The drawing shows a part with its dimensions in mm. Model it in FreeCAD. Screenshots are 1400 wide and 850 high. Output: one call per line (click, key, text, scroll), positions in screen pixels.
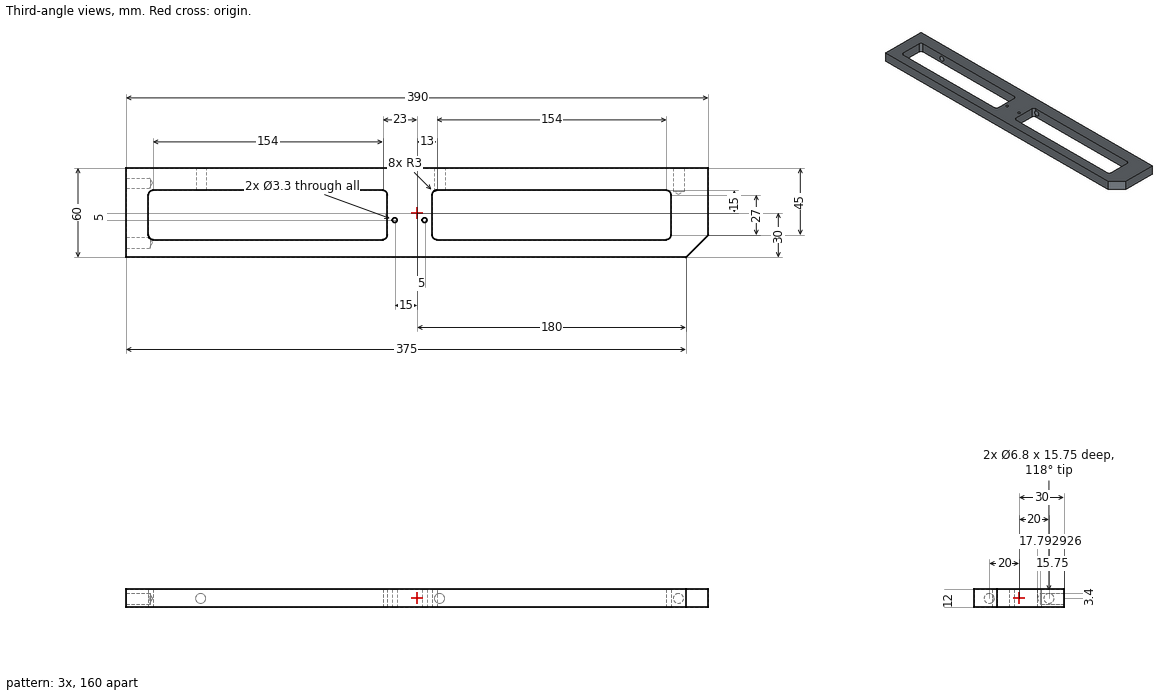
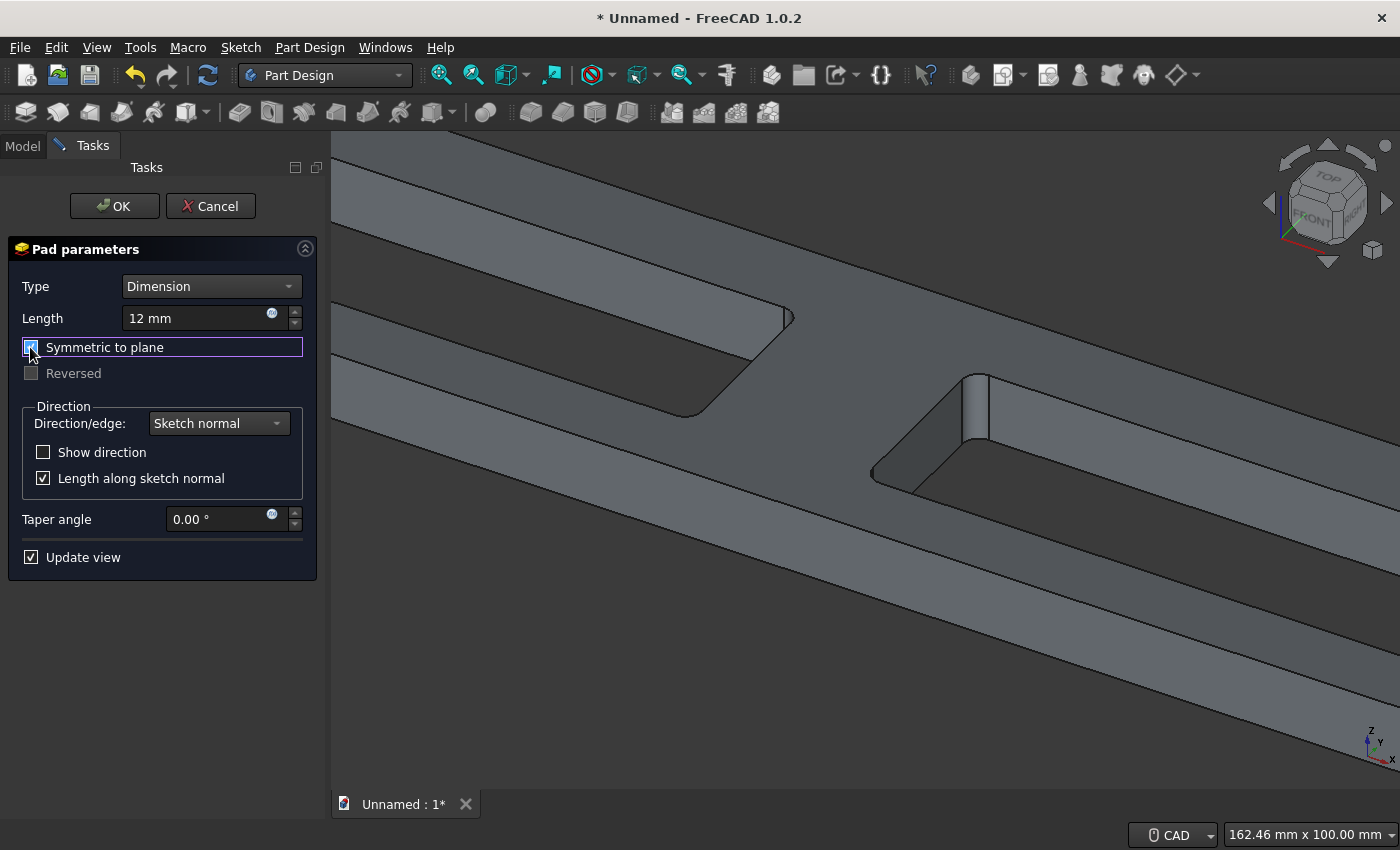
click(115, 206)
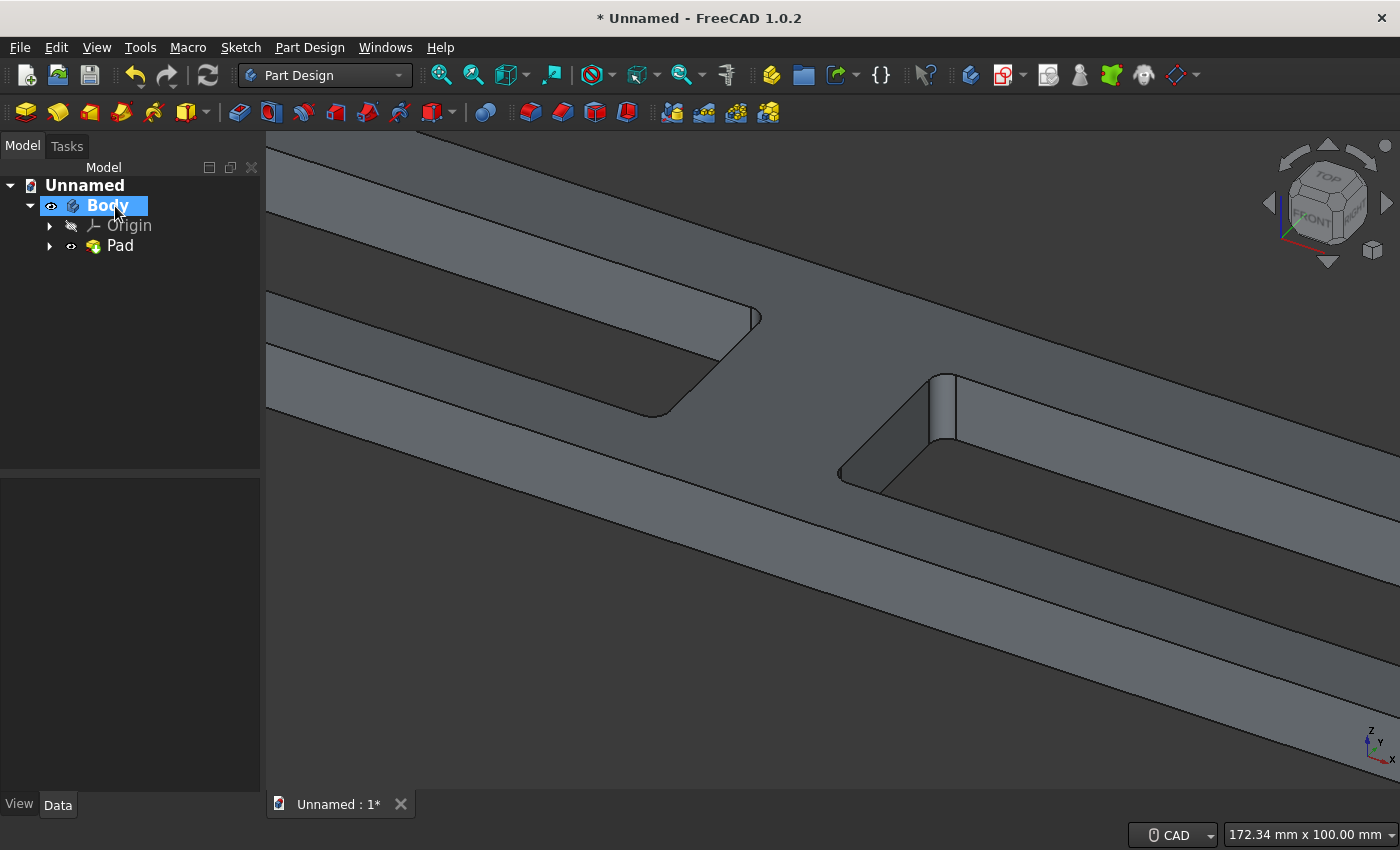
key(v)
key(f)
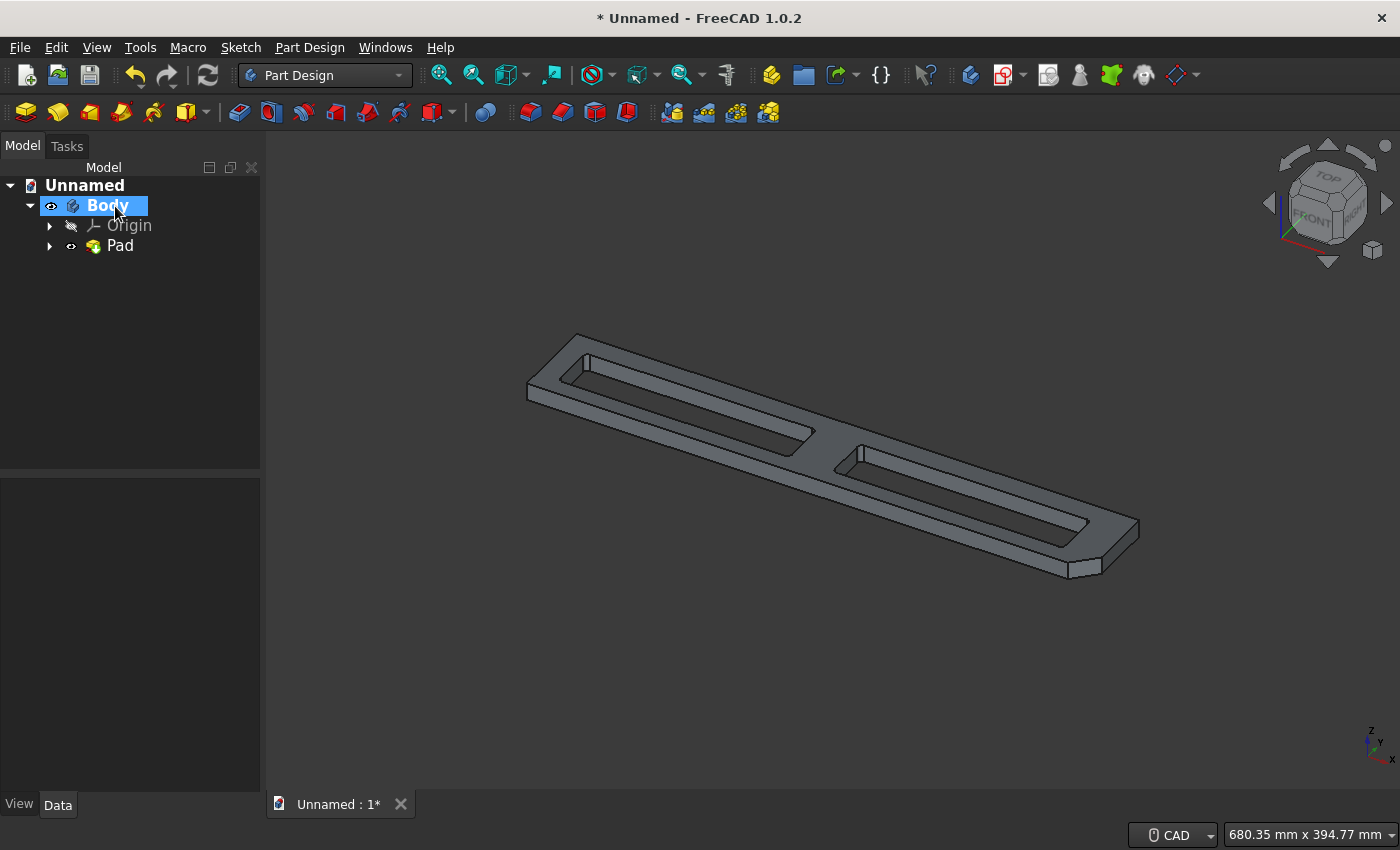
key(6)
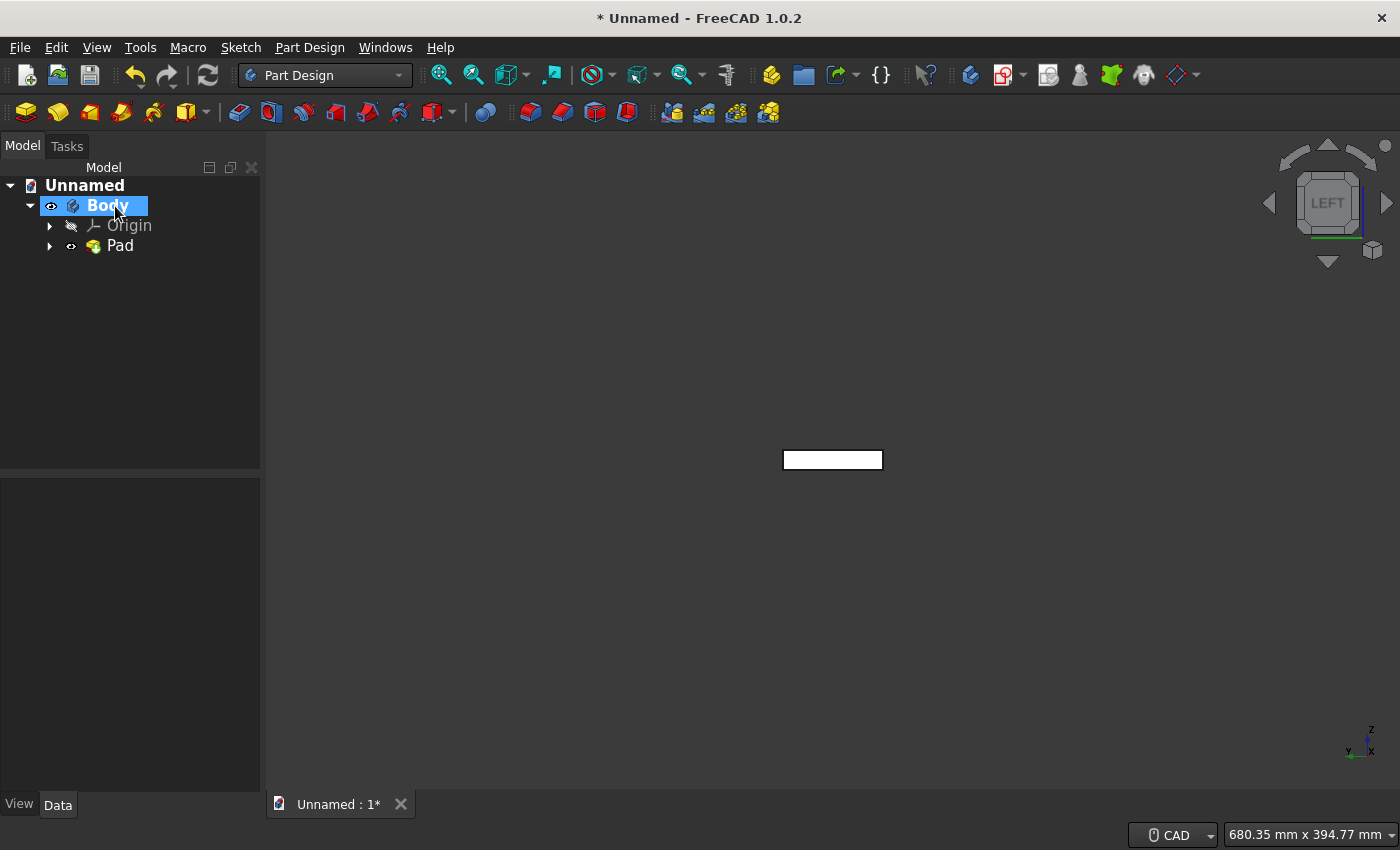
key(v)
key(f)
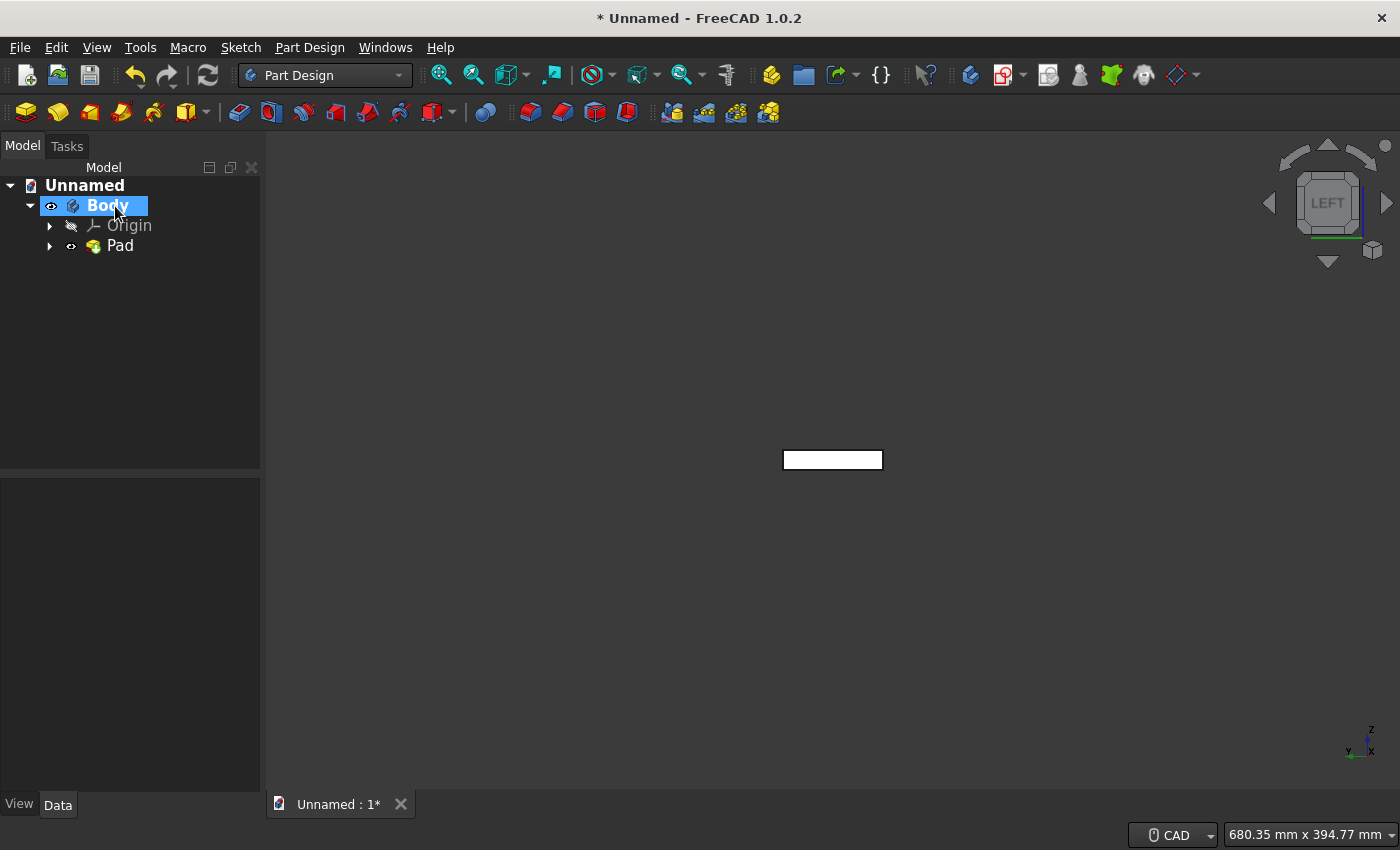
click(804, 459)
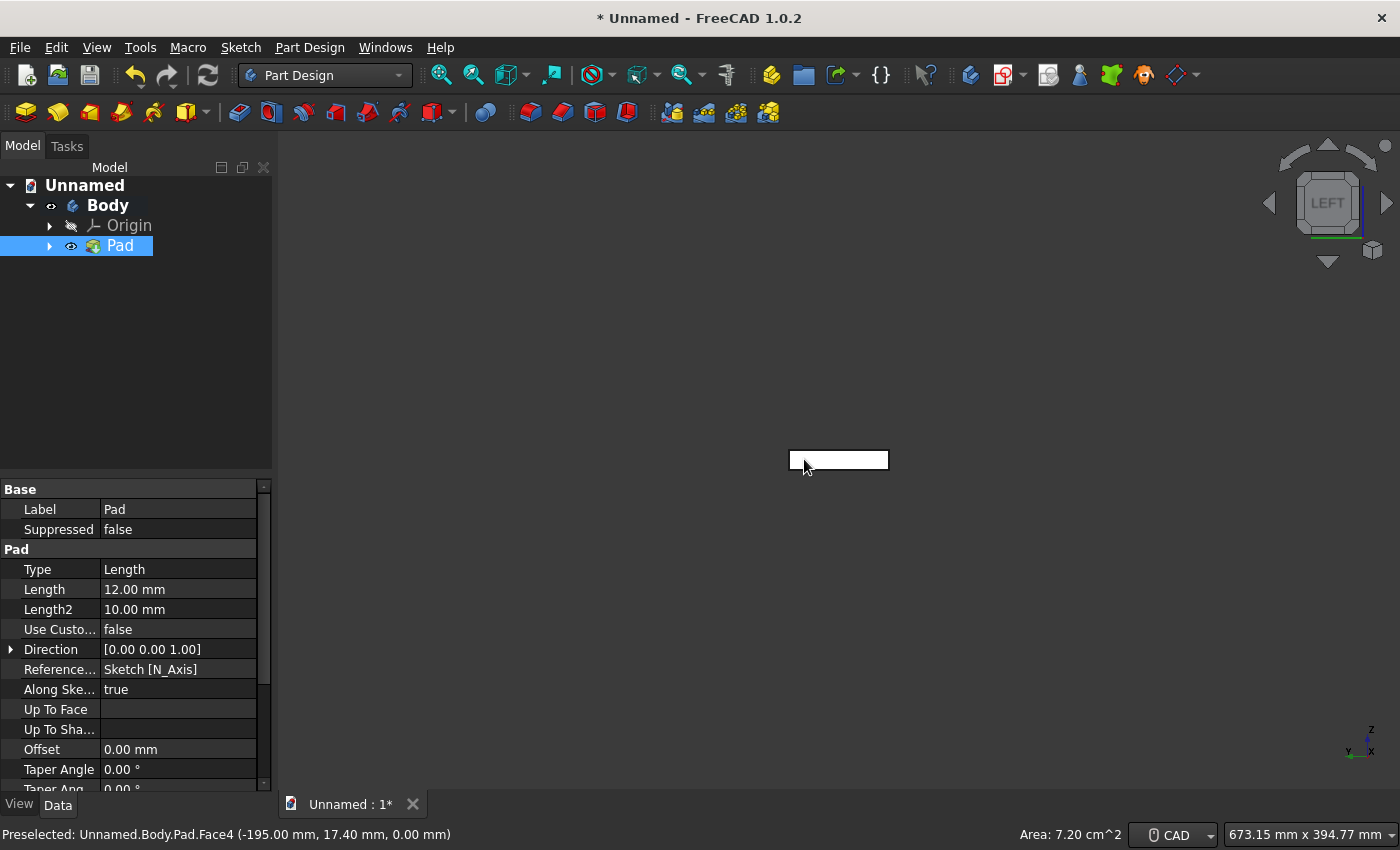
click(1004, 76)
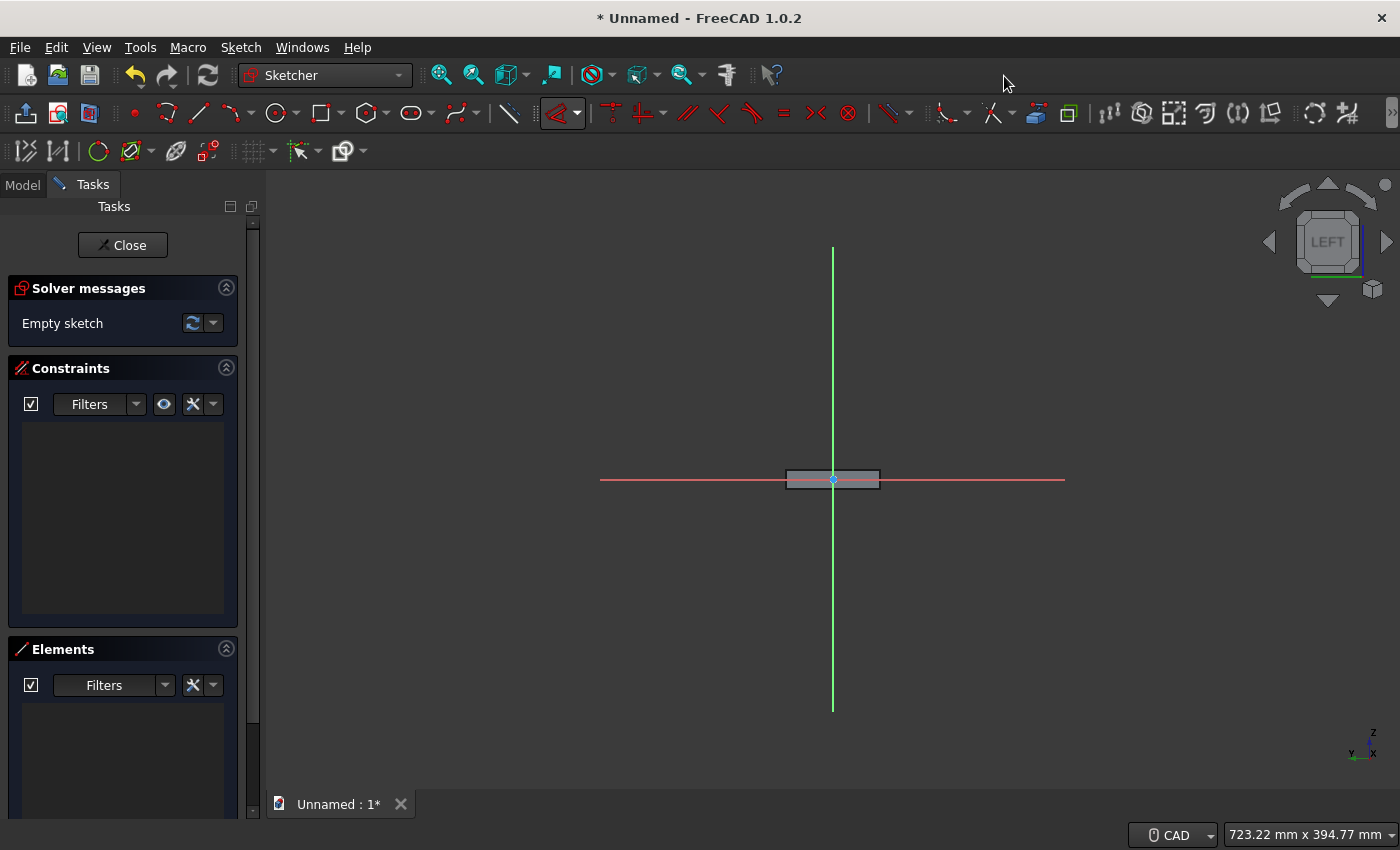
scroll(842, 479, up, 11)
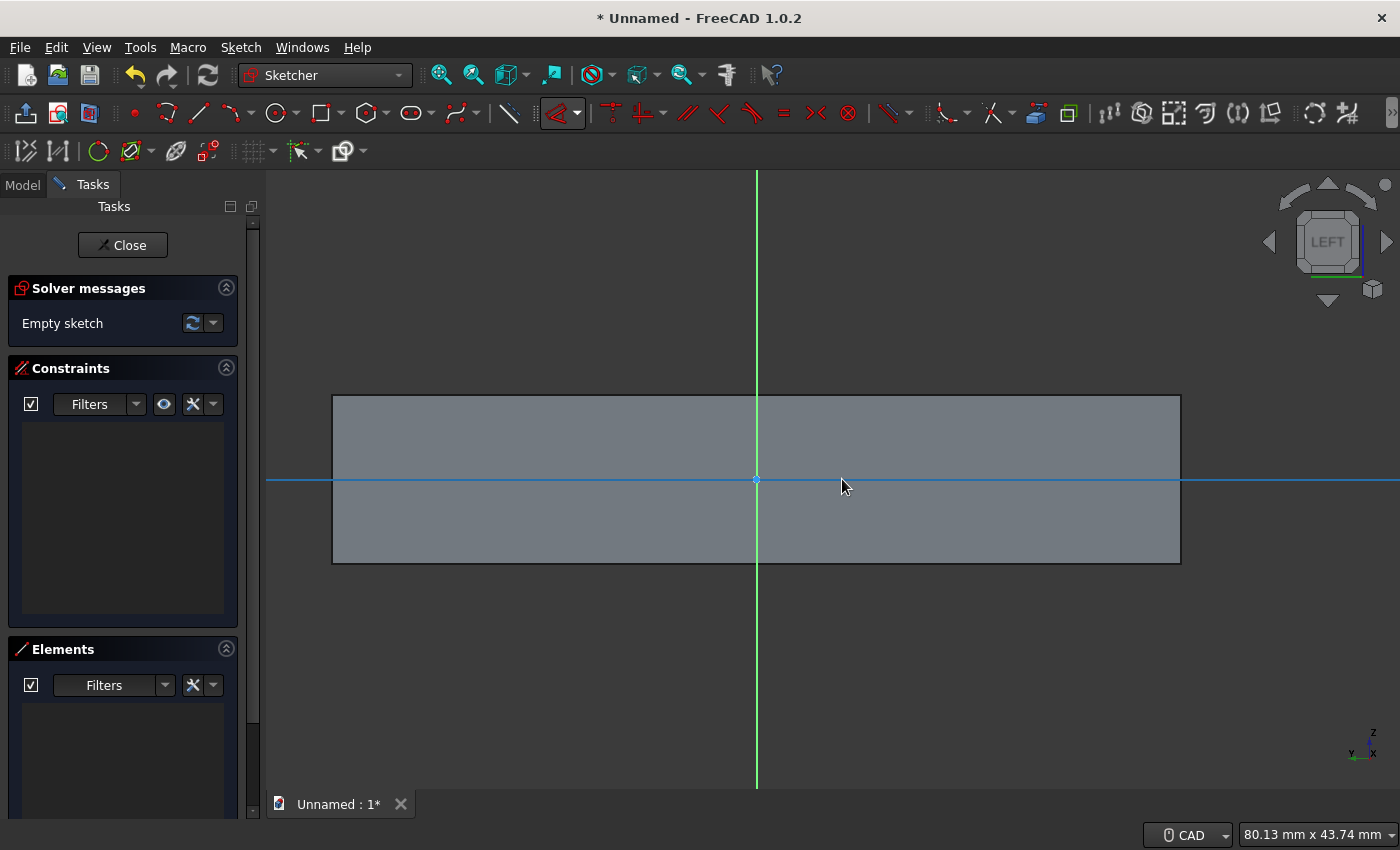
click(276, 114)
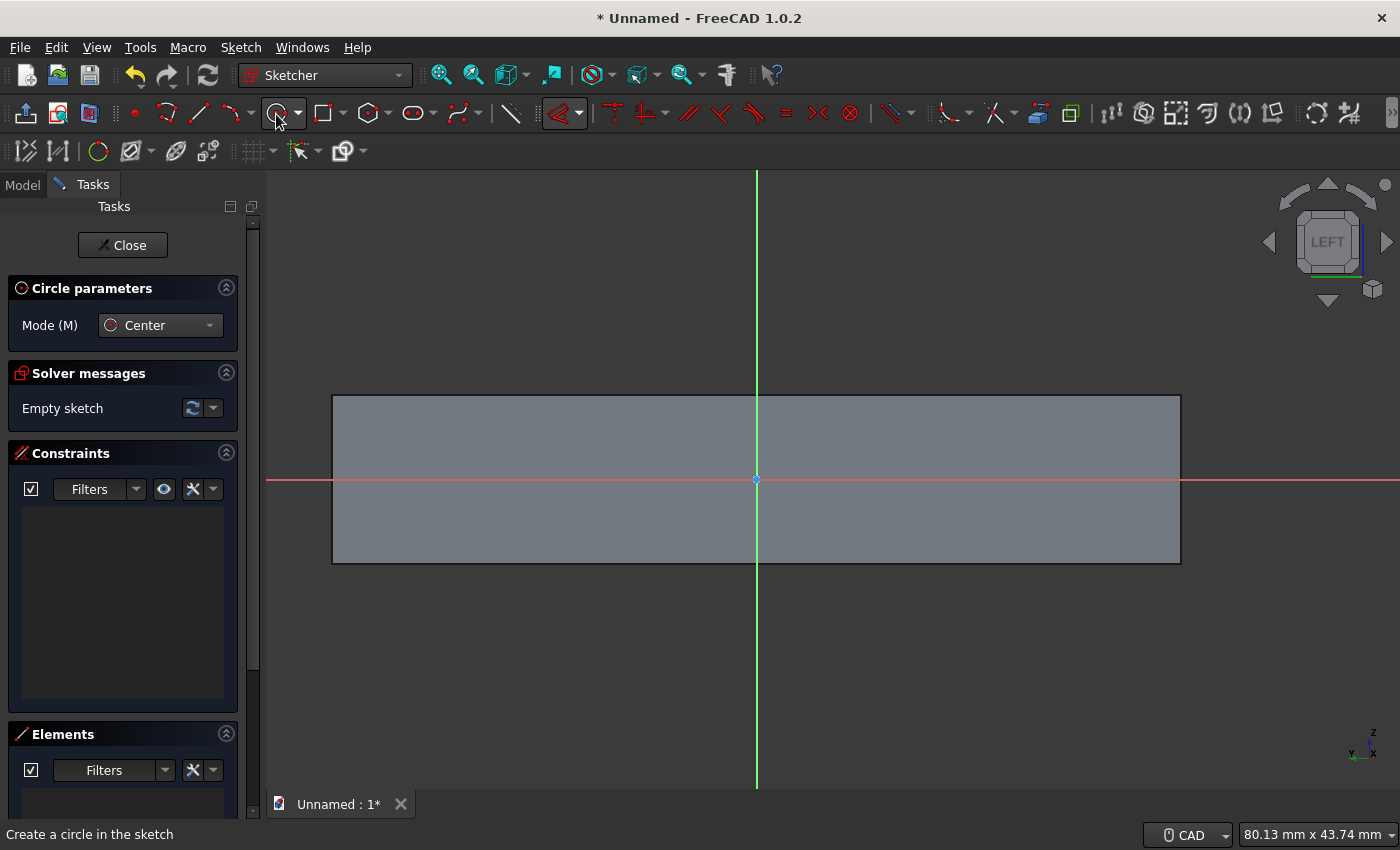
click(474, 480)
move(508, 445)